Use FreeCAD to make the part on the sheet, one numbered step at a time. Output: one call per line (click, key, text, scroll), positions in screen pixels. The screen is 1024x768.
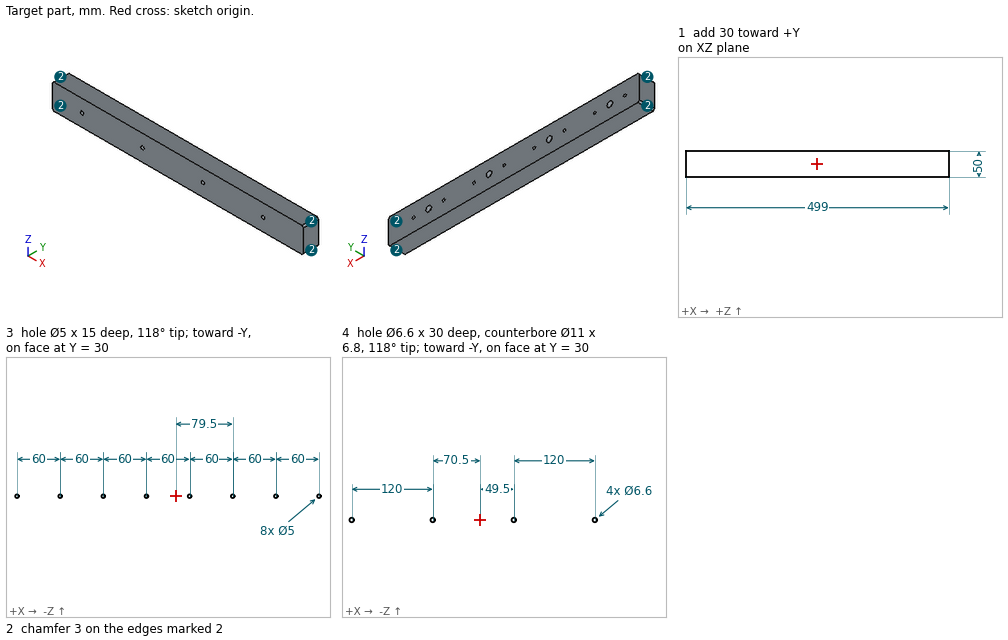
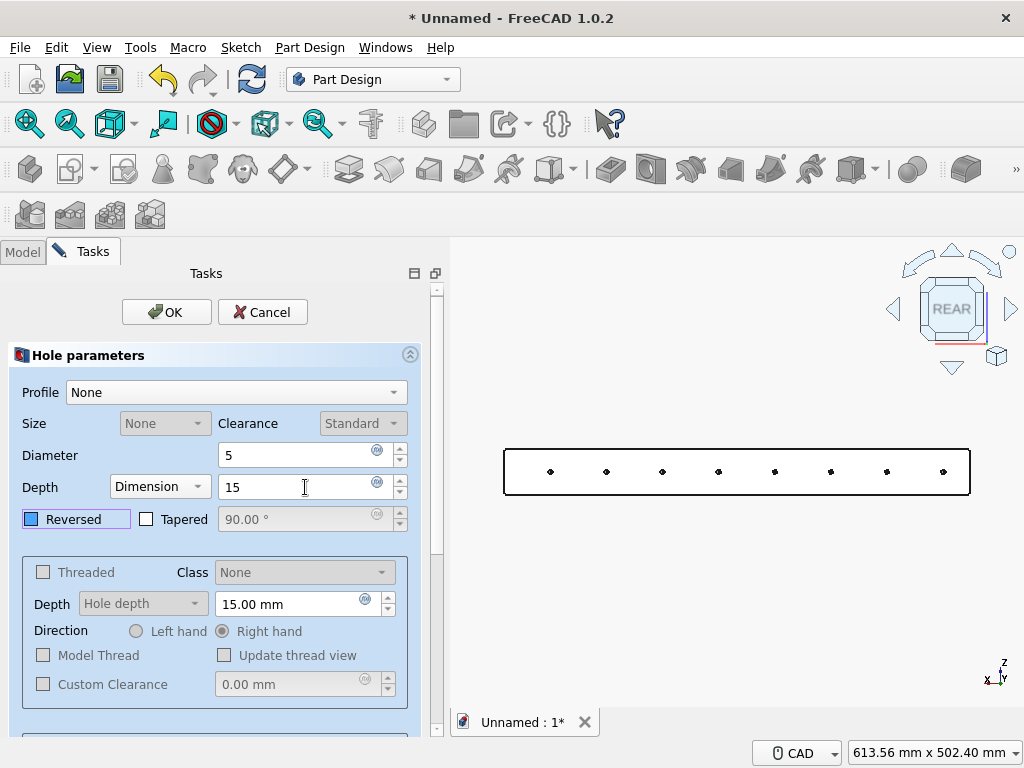
click(167, 312)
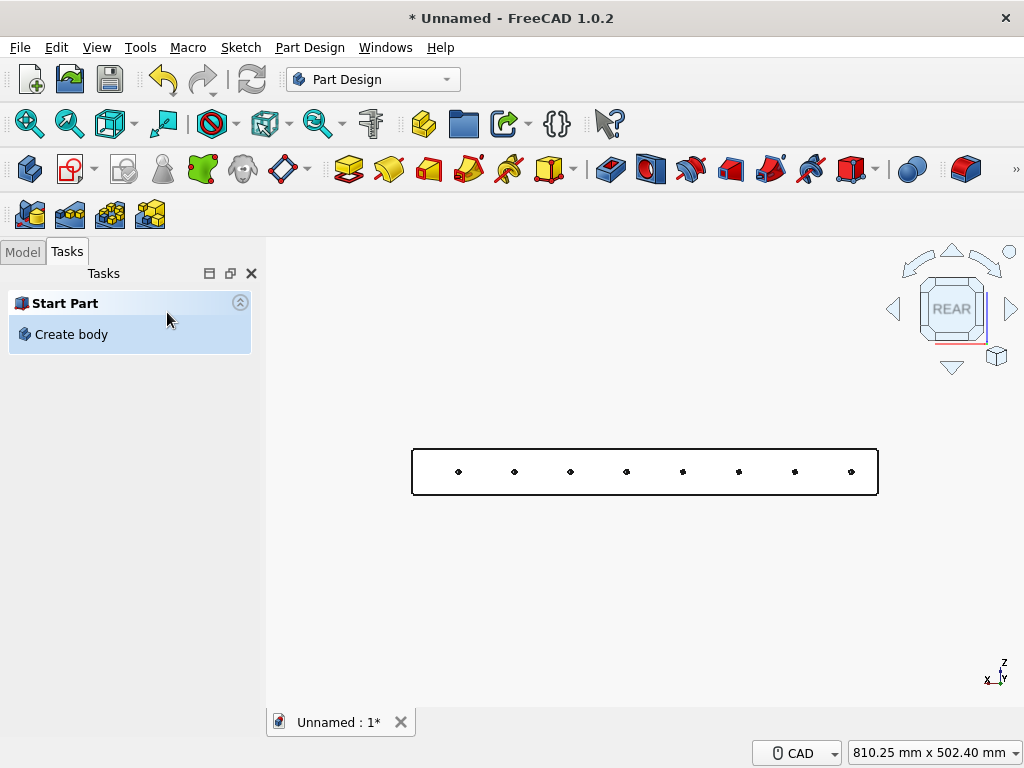
click(712, 471)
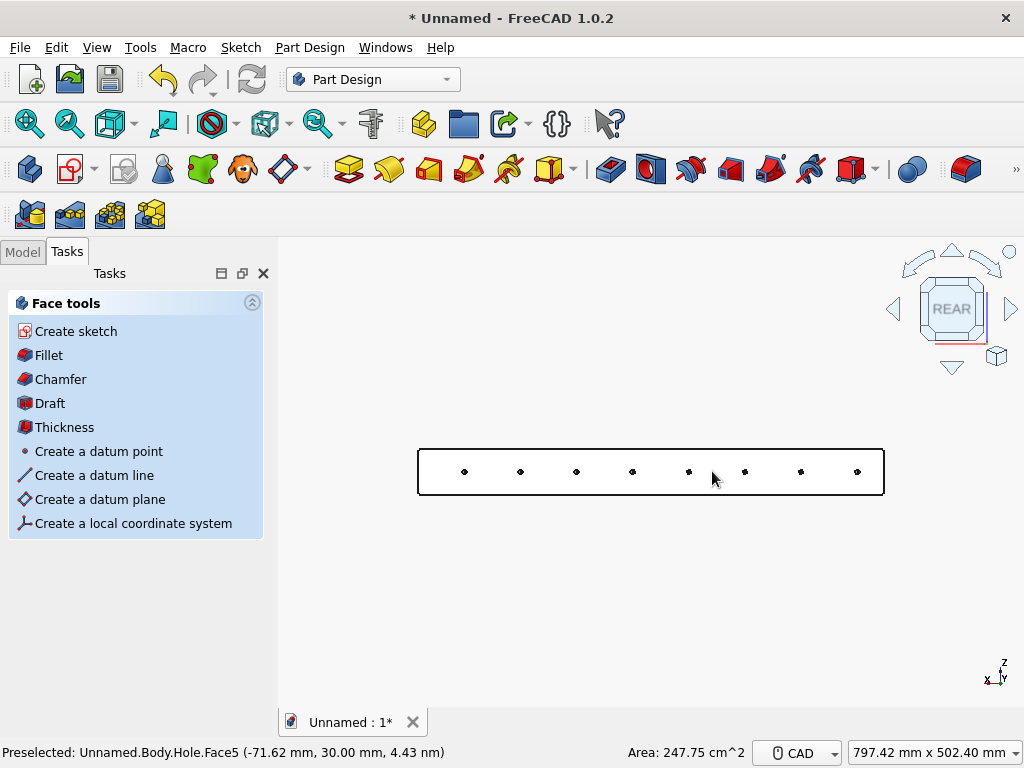
click(70, 170)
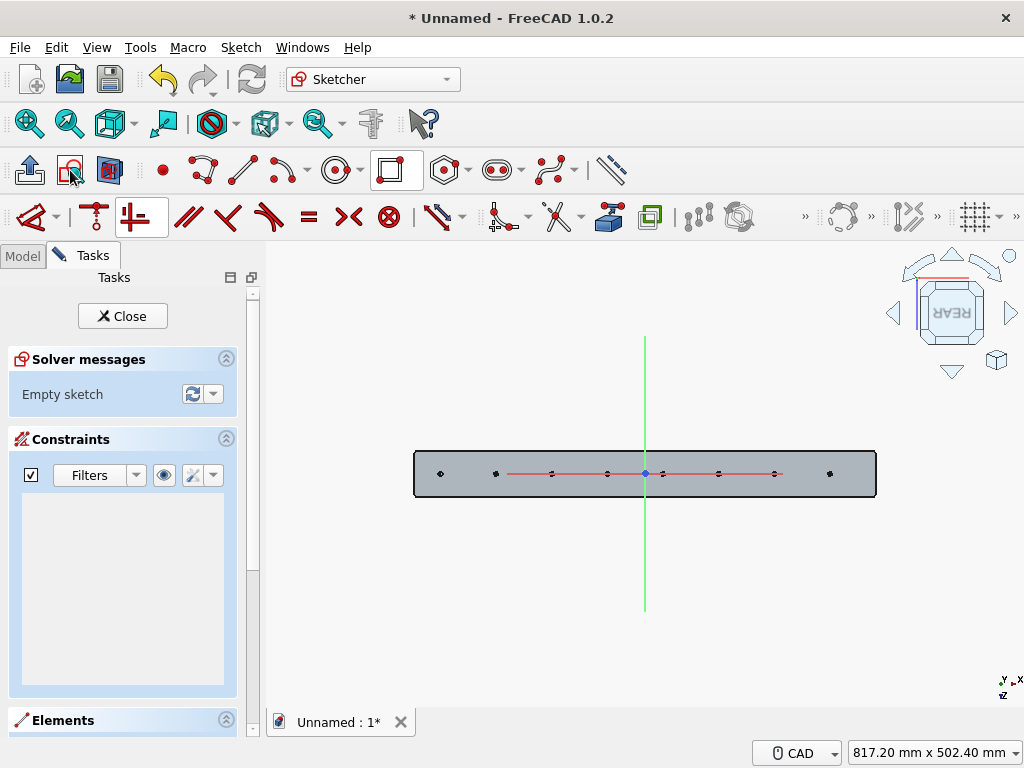
key(g)
key(c)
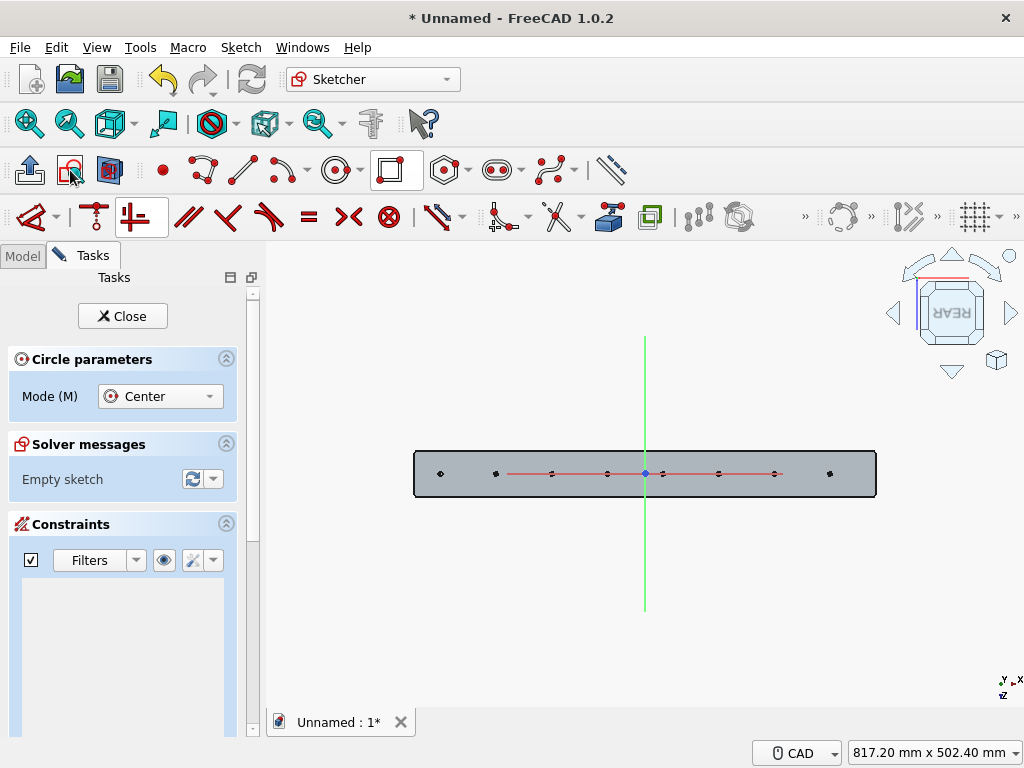
scroll(802, 474, up, 11)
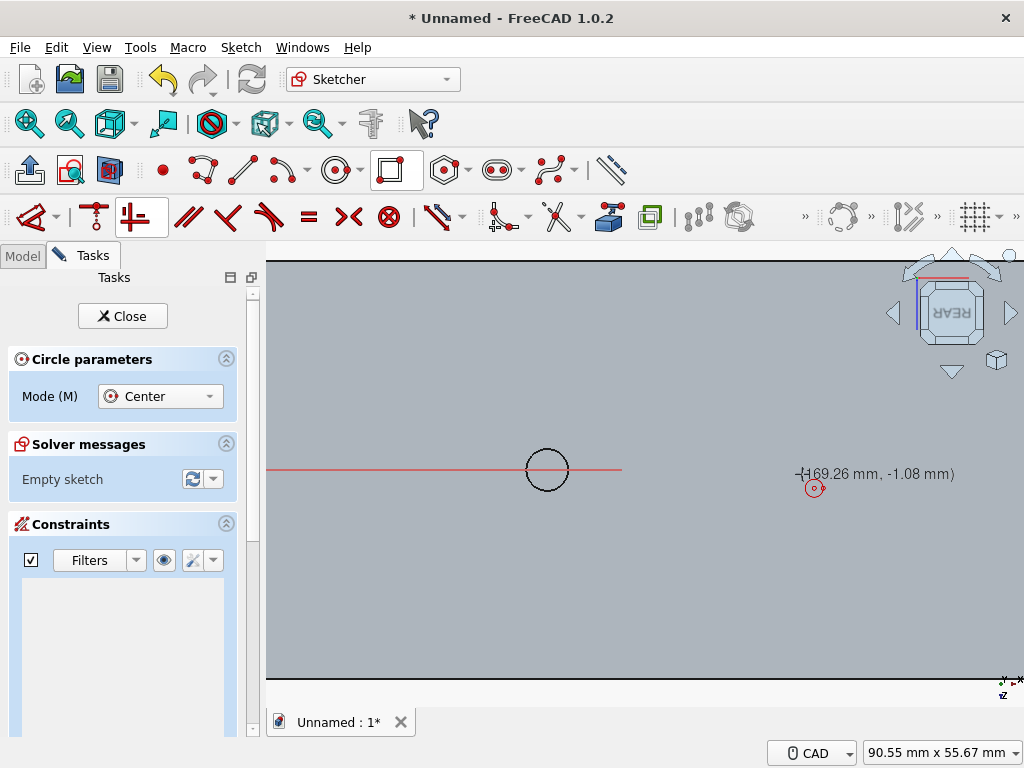
scroll(778, 475, down, 10)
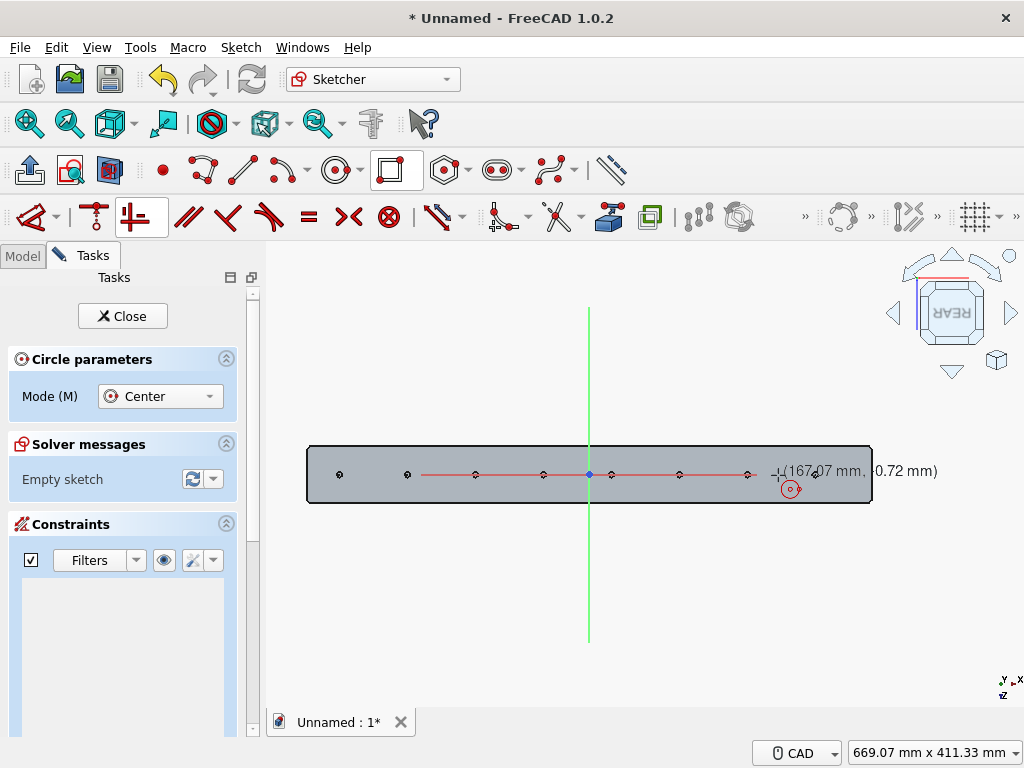
click(781, 475)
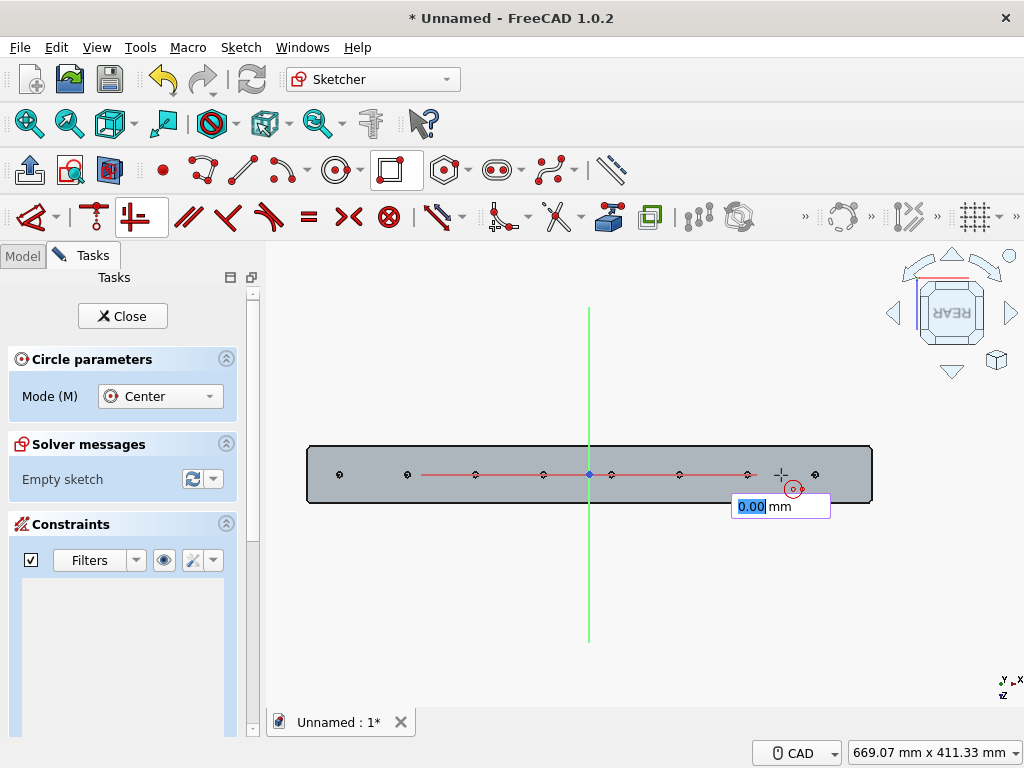
scroll(780, 478, up, 8)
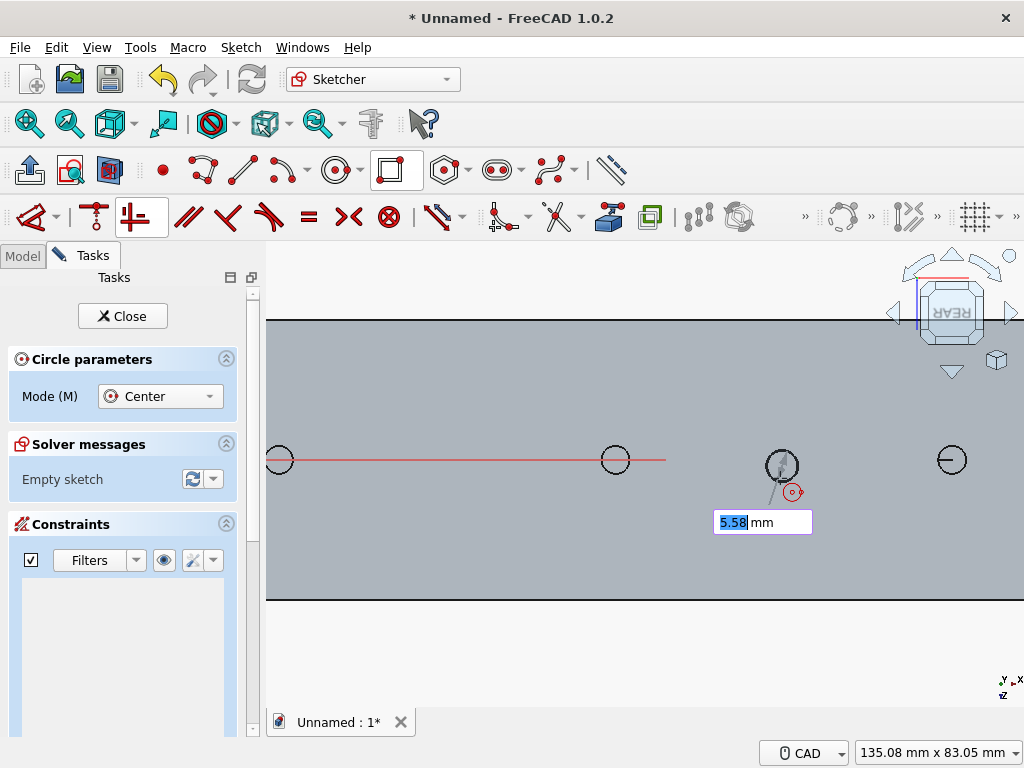
click(778, 477)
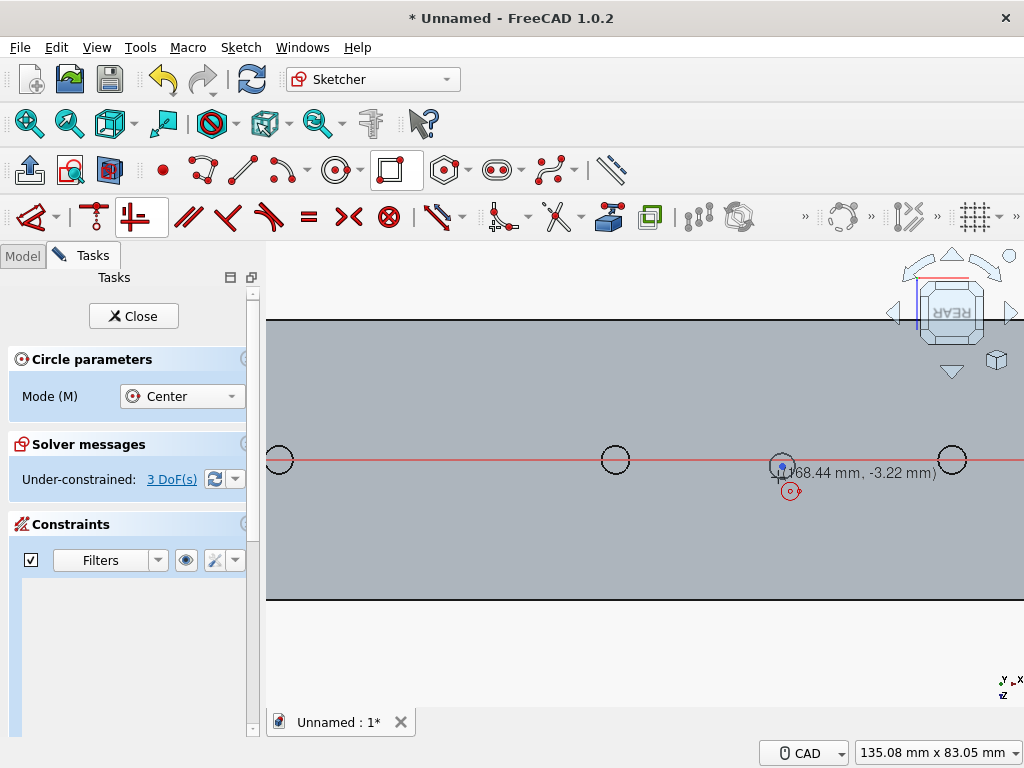
scroll(780, 478, down, 8)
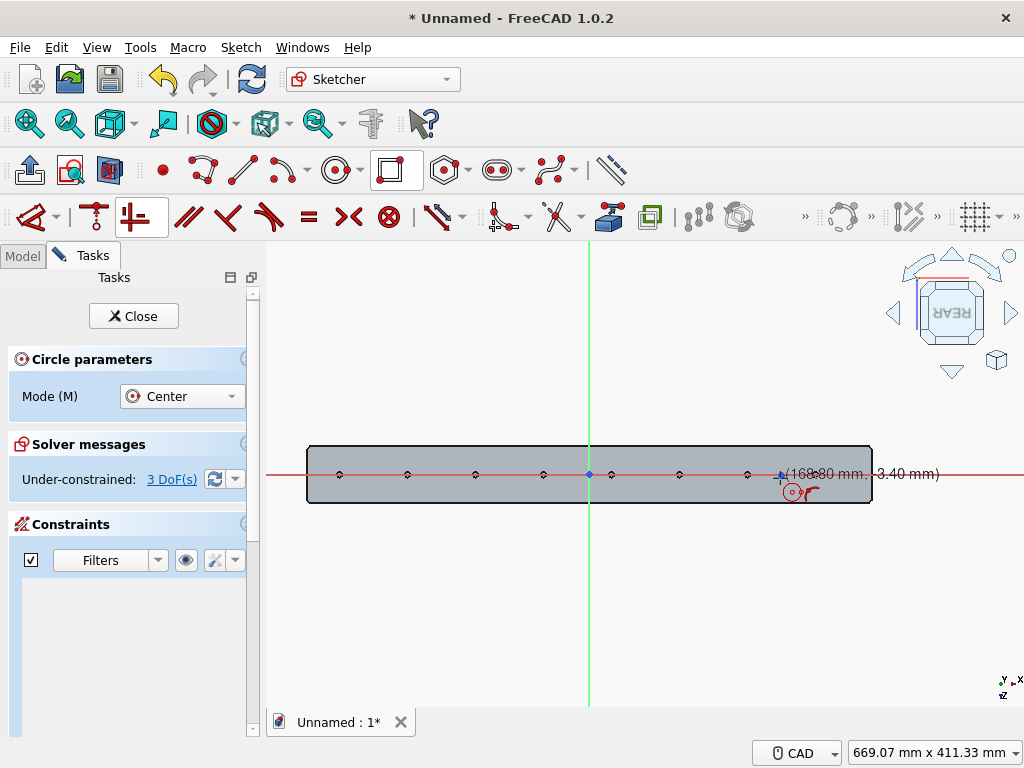
scroll(645, 475, up, 10)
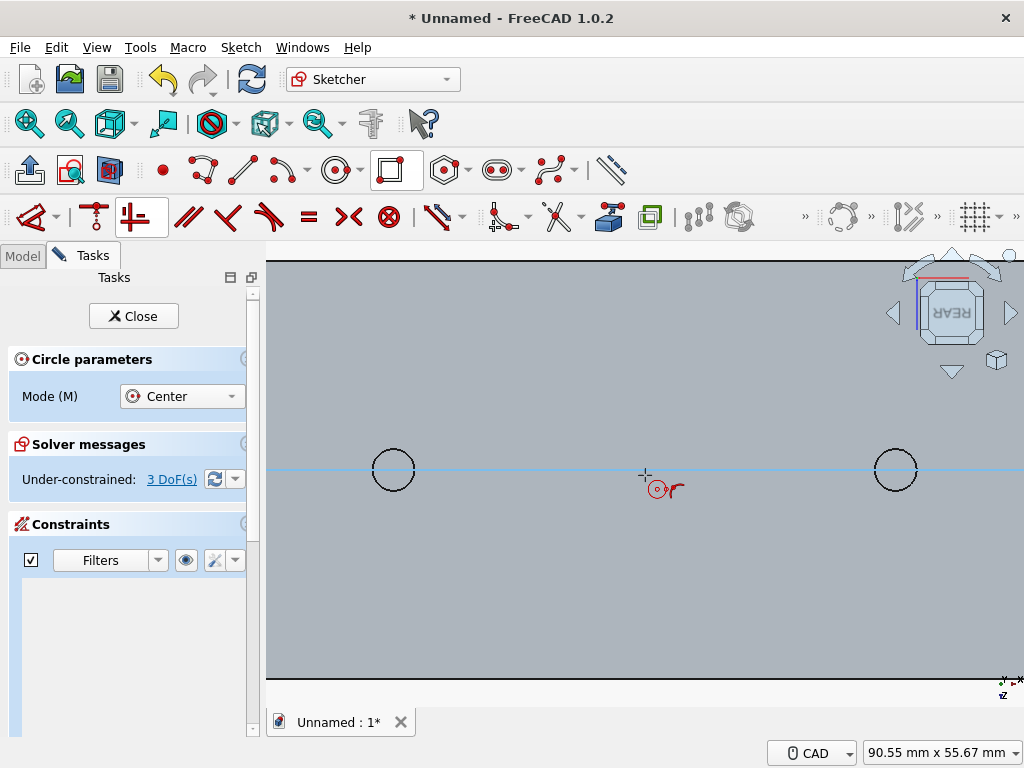
scroll(644, 475, down, 10)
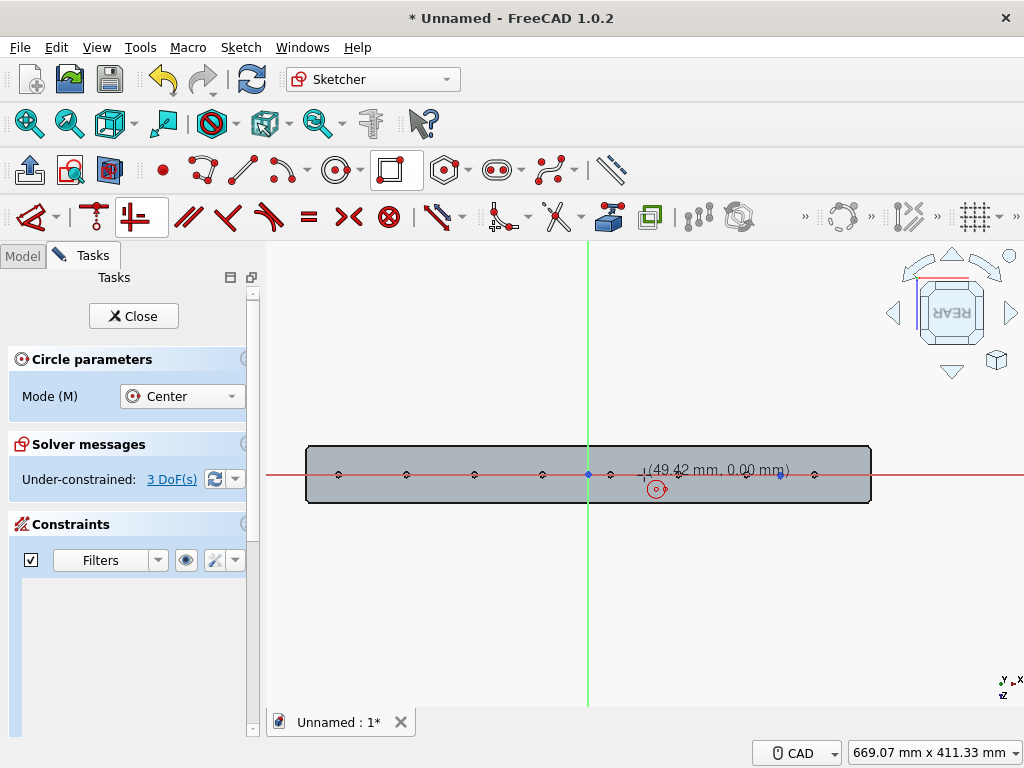
click(645, 475)